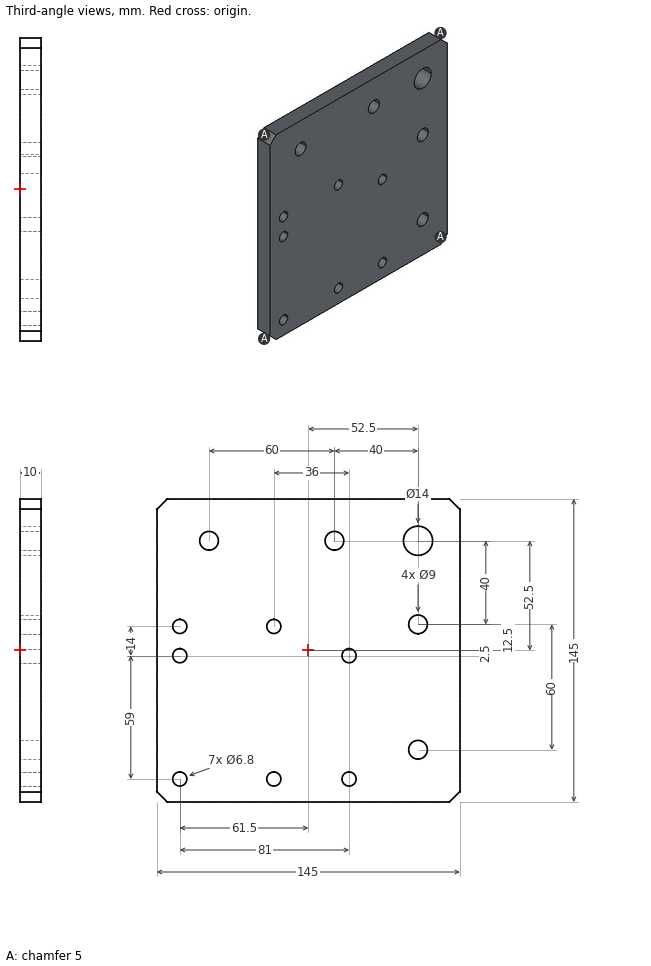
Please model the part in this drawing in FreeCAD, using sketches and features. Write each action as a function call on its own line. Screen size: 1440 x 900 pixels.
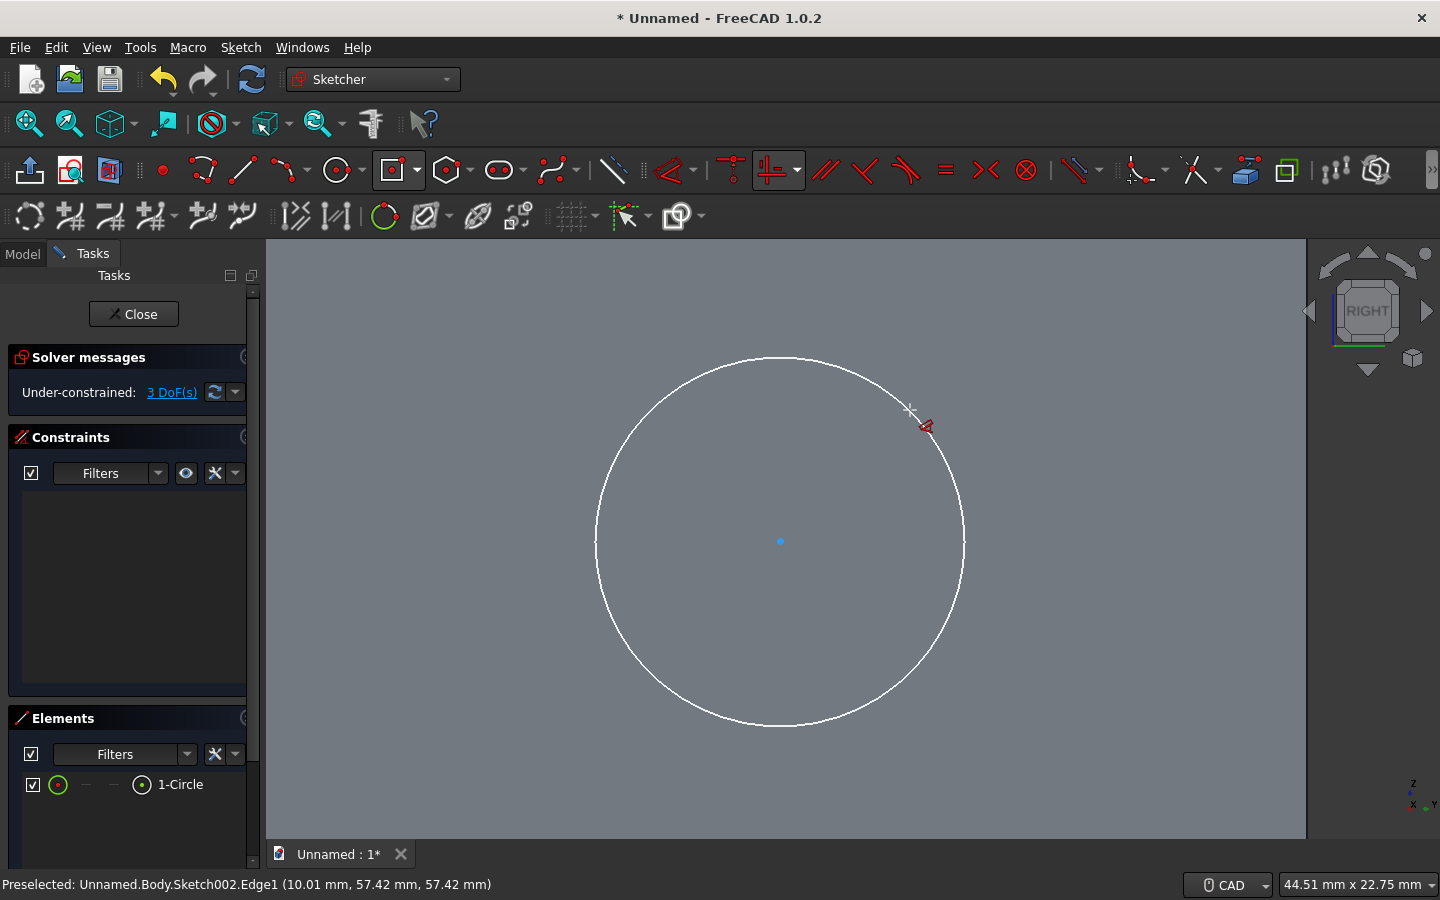
click(910, 411)
click(933, 388)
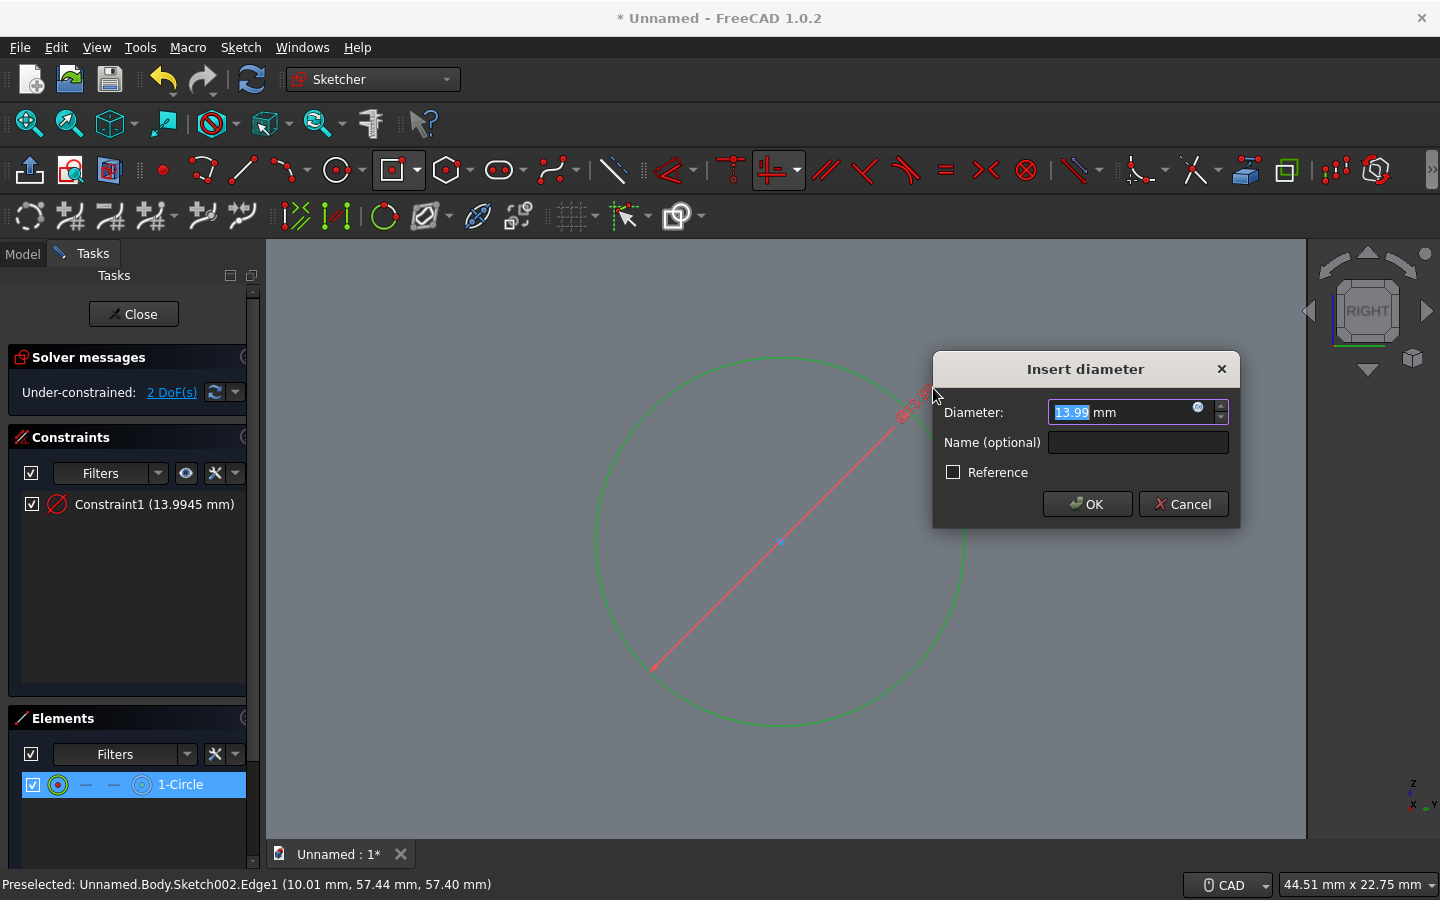
text(14)
key(Return)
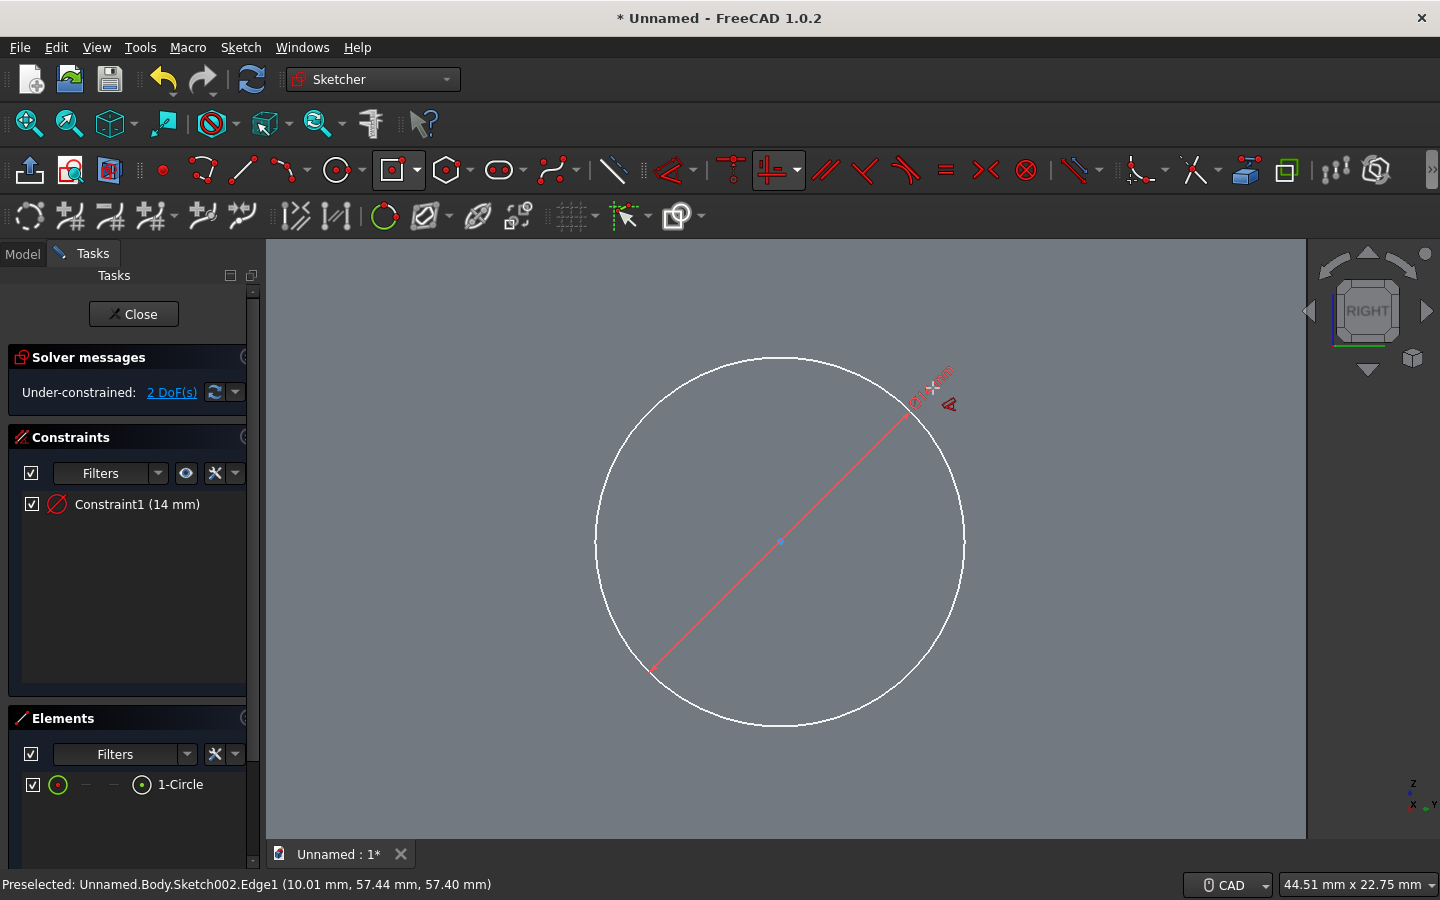
click(780, 542)
click(537, 508)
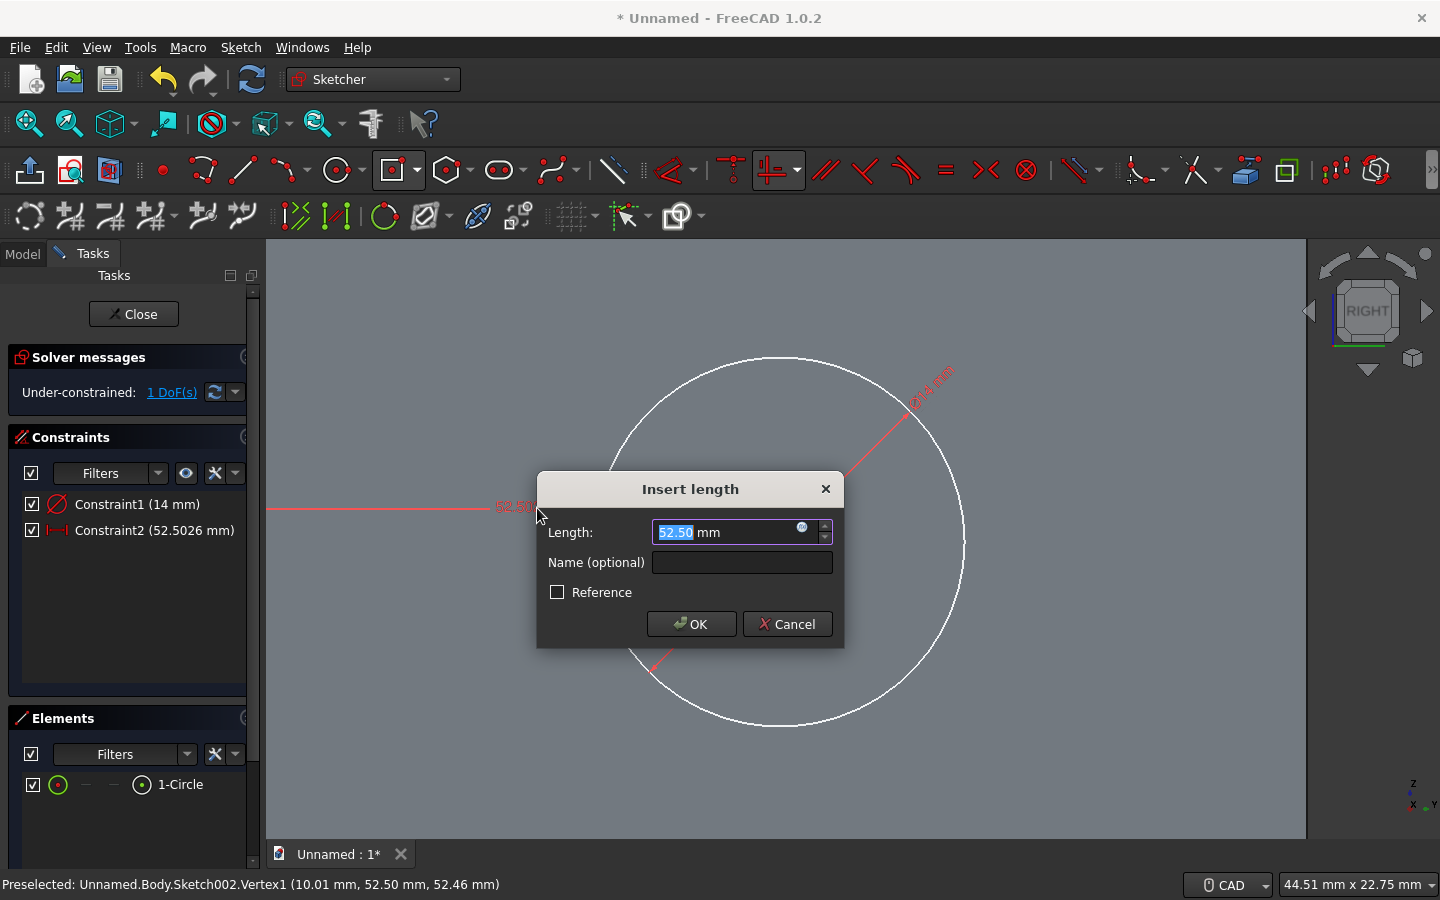
text(52.5)
key(Return)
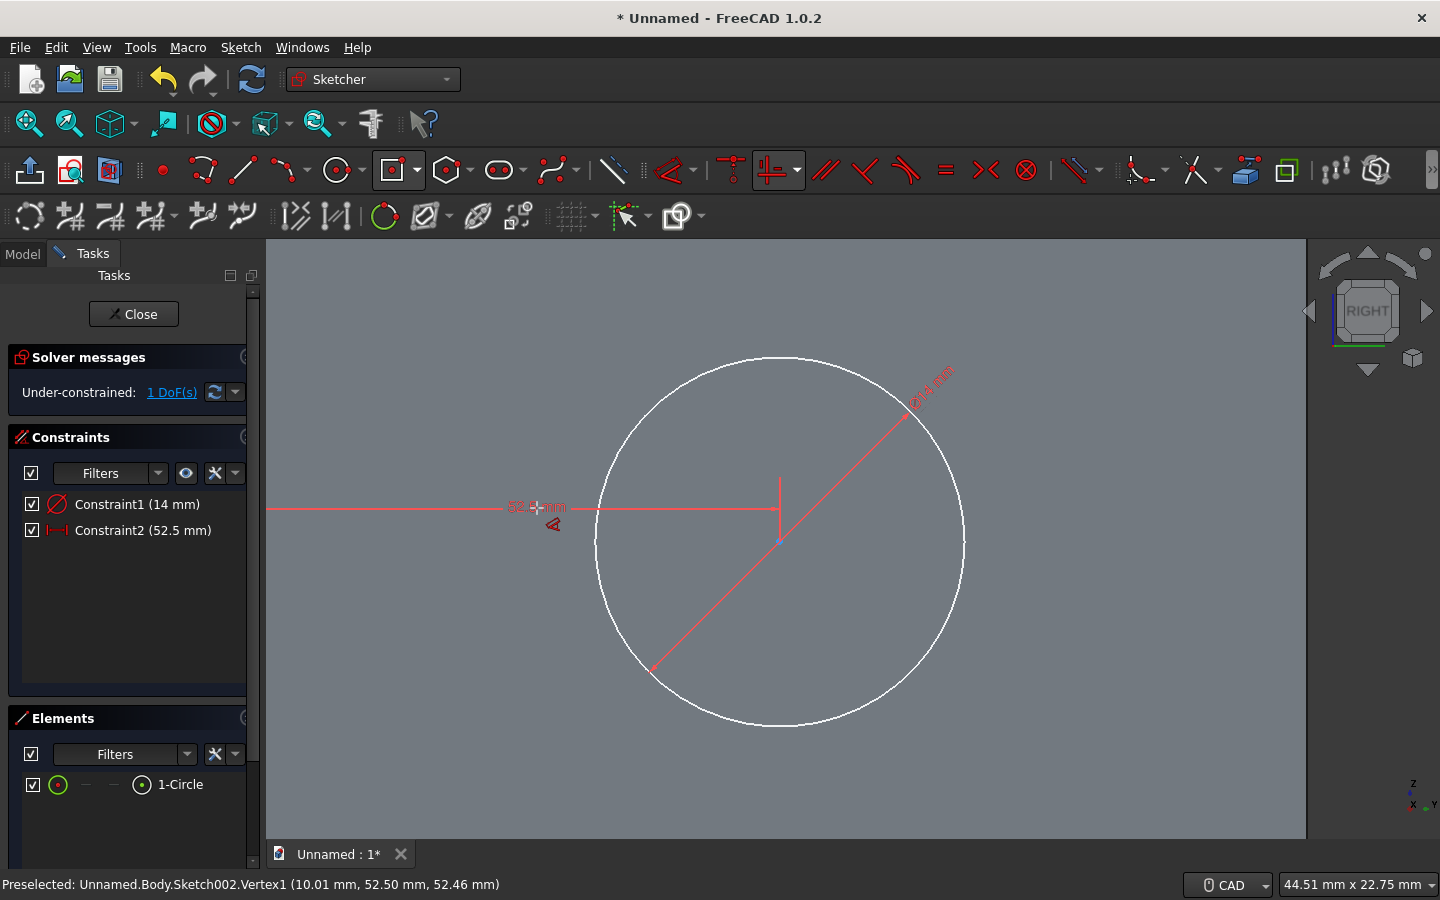
click(780, 542)
click(814, 677)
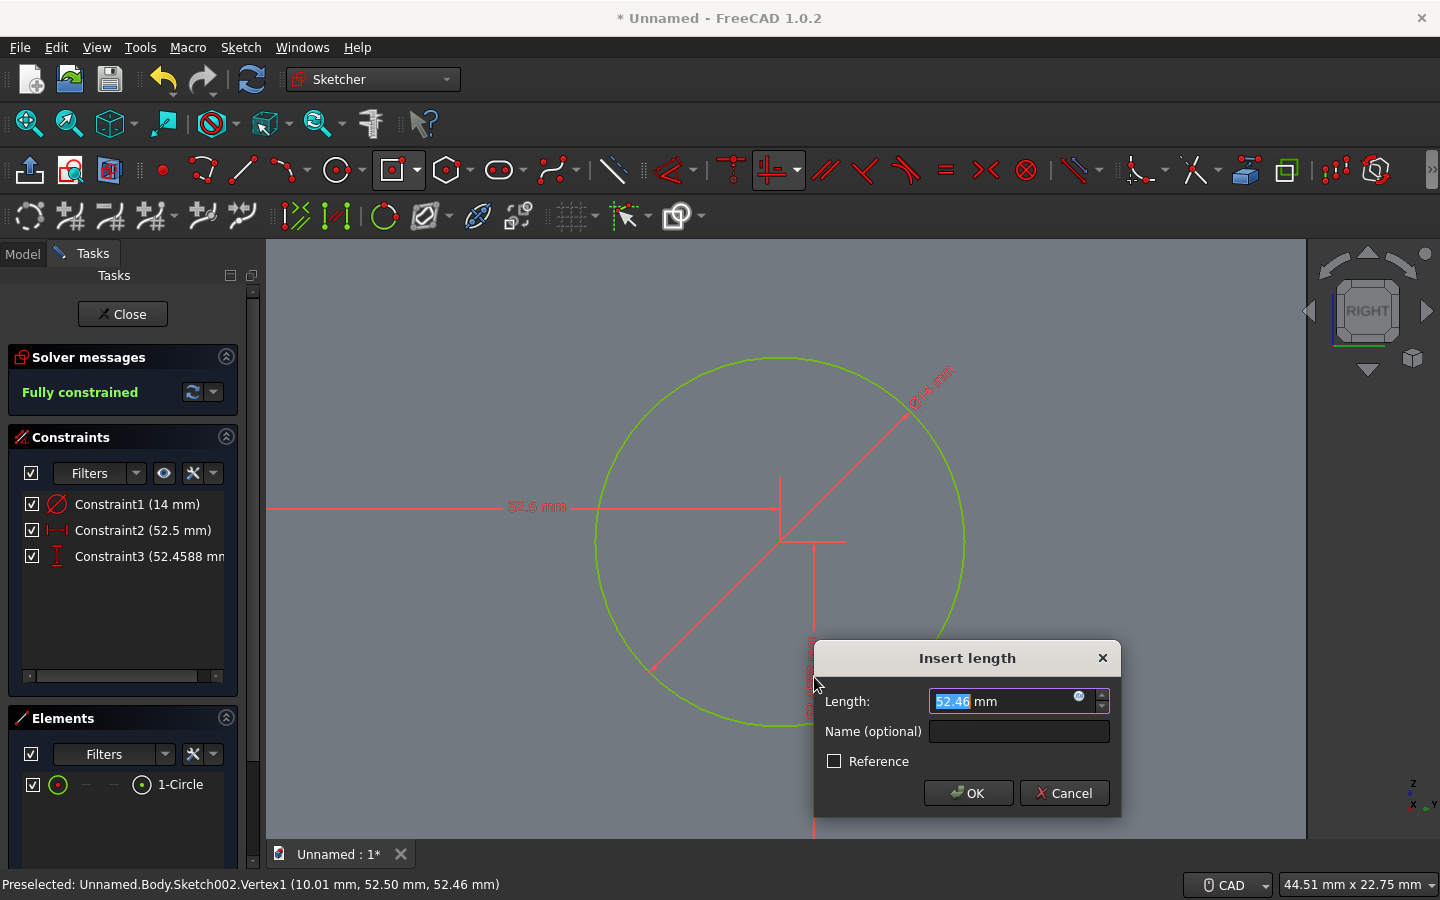
text(52.5)
key(Return)
key(Escape)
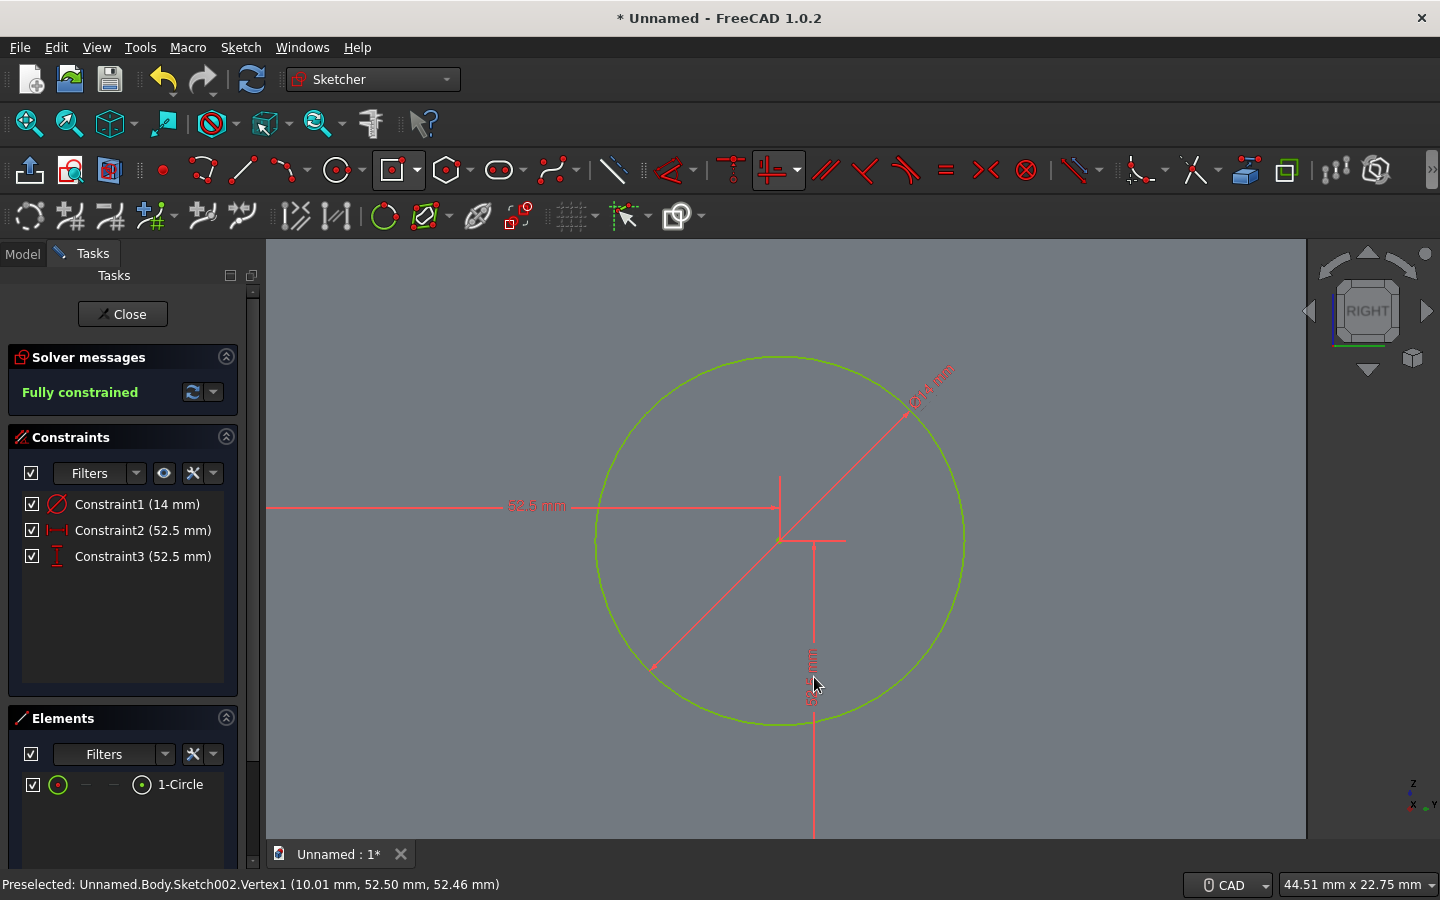
click(123, 314)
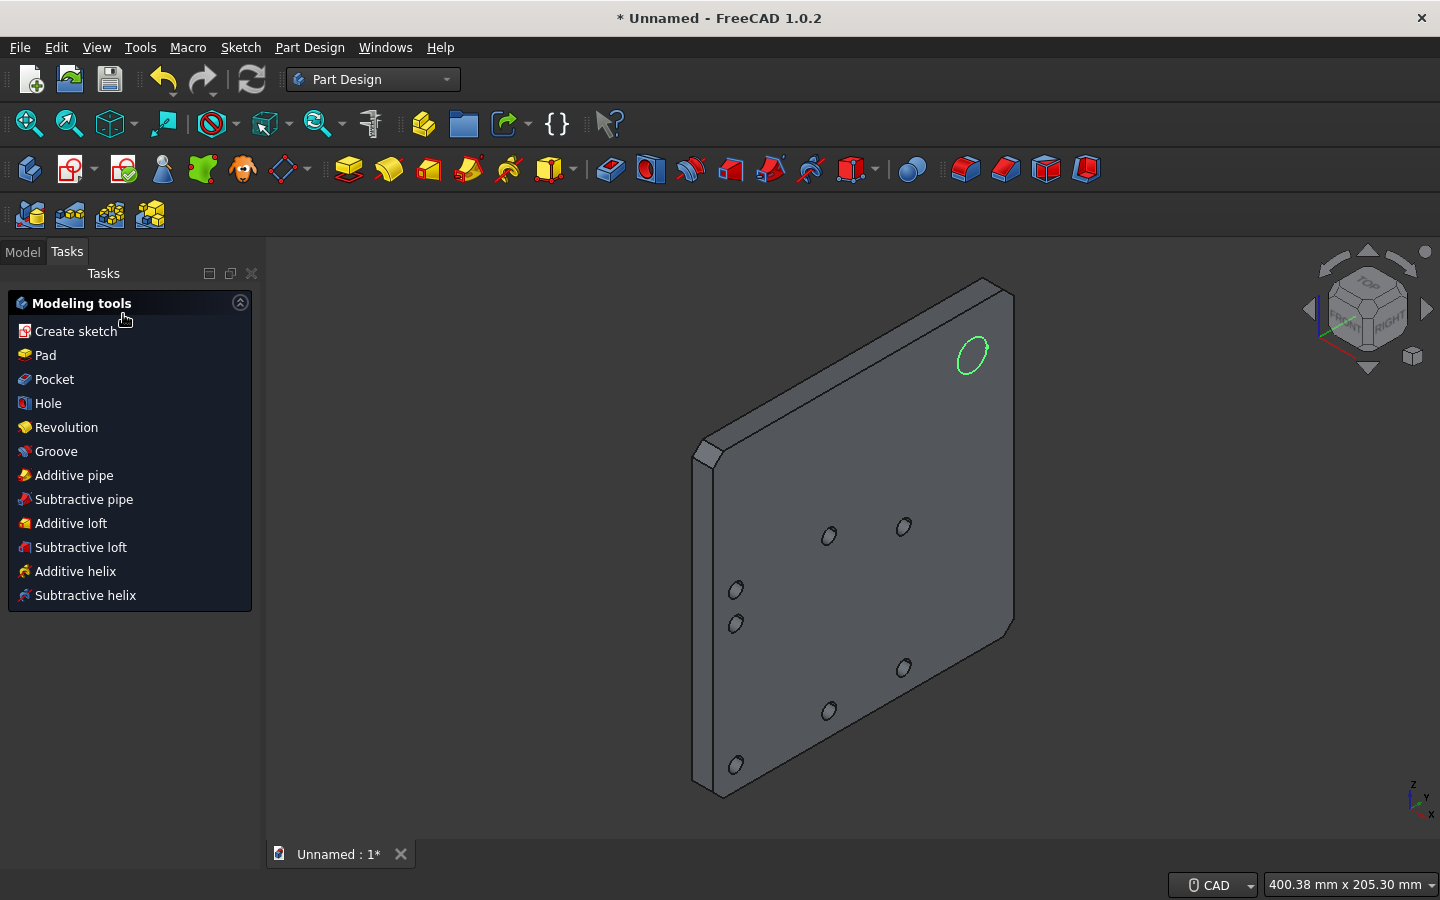
click(612, 170)